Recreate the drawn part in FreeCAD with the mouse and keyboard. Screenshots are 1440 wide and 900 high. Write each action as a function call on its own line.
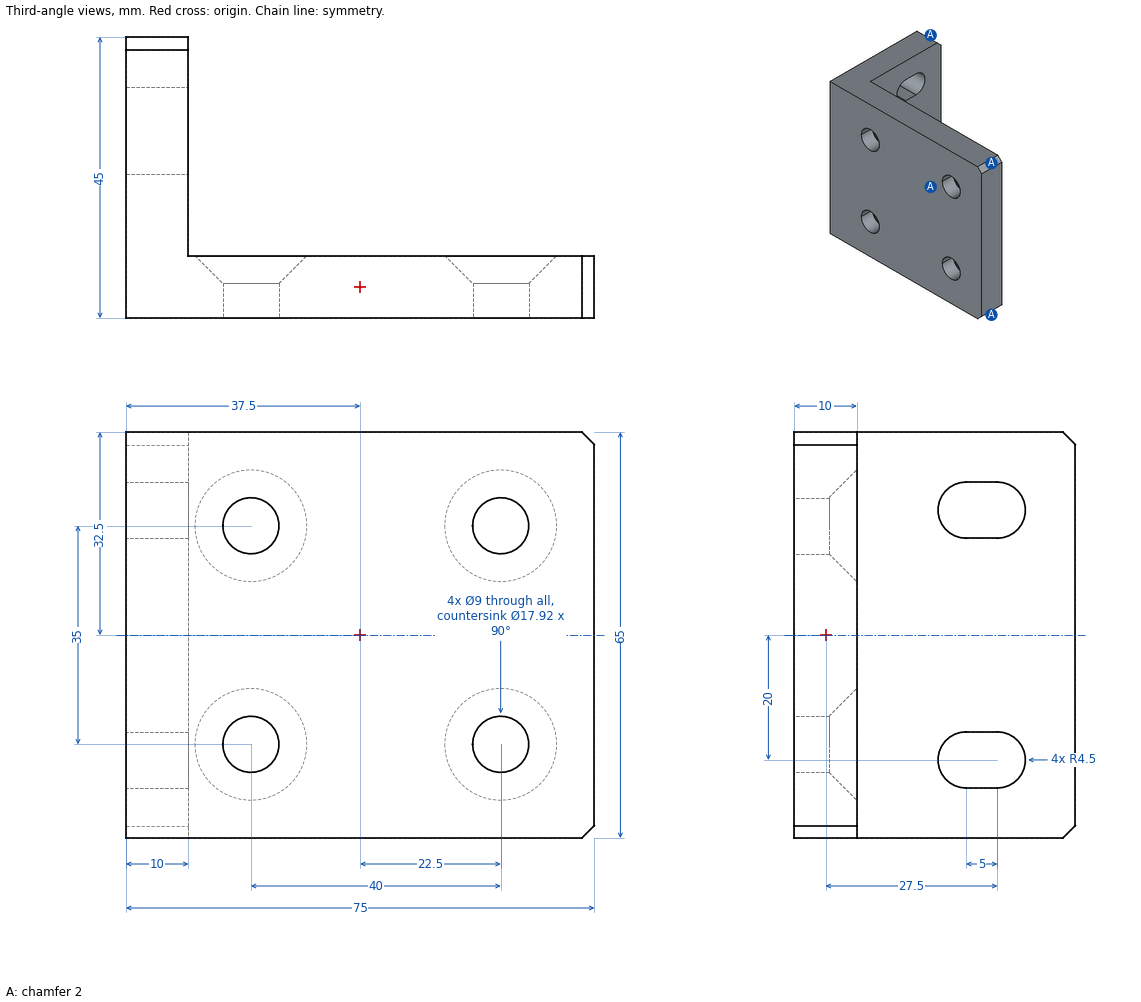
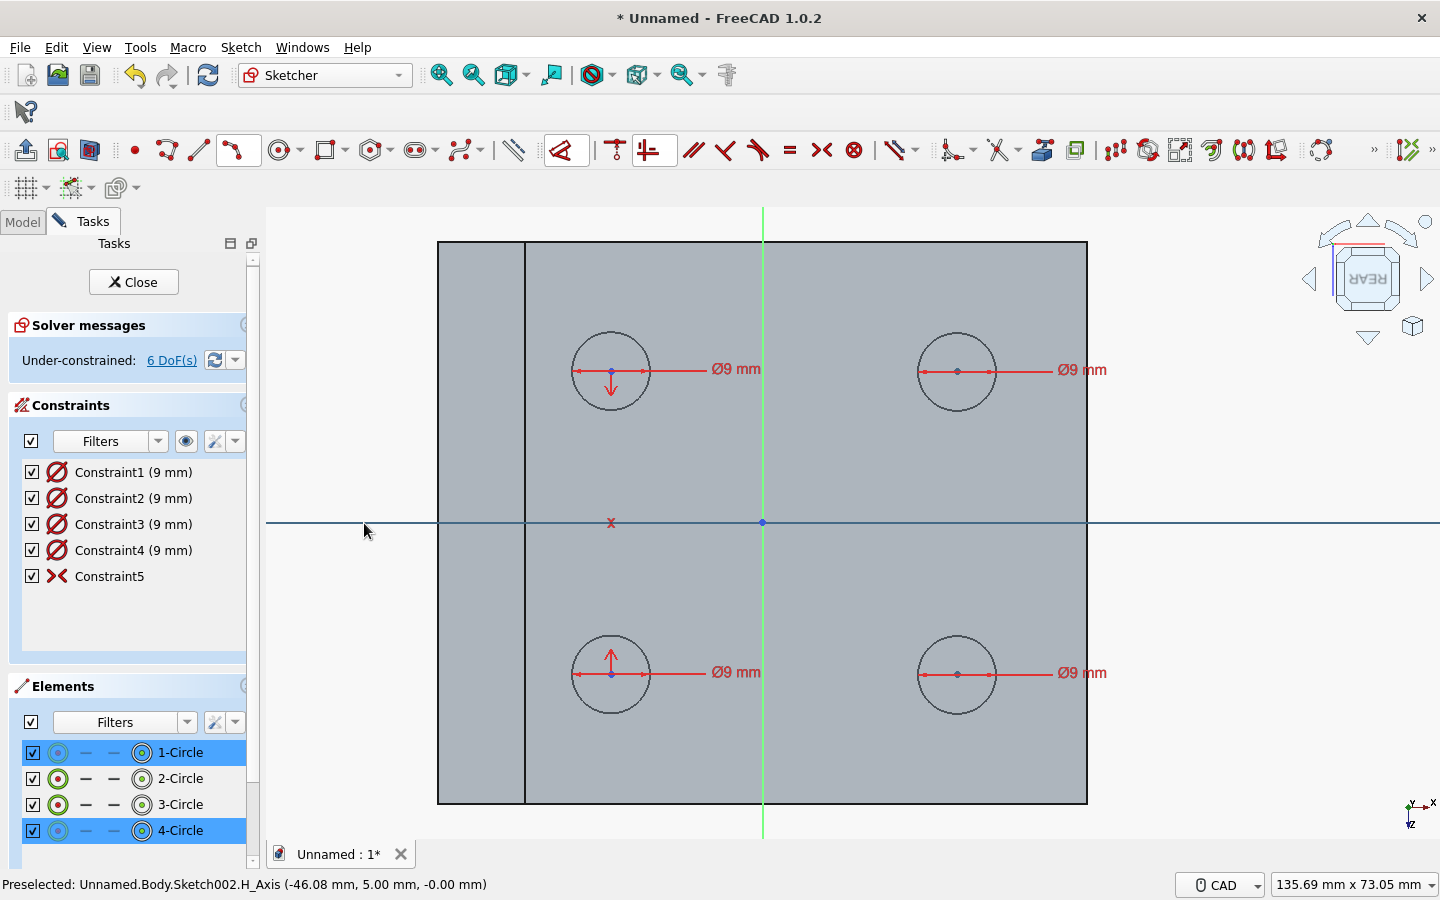
key(s)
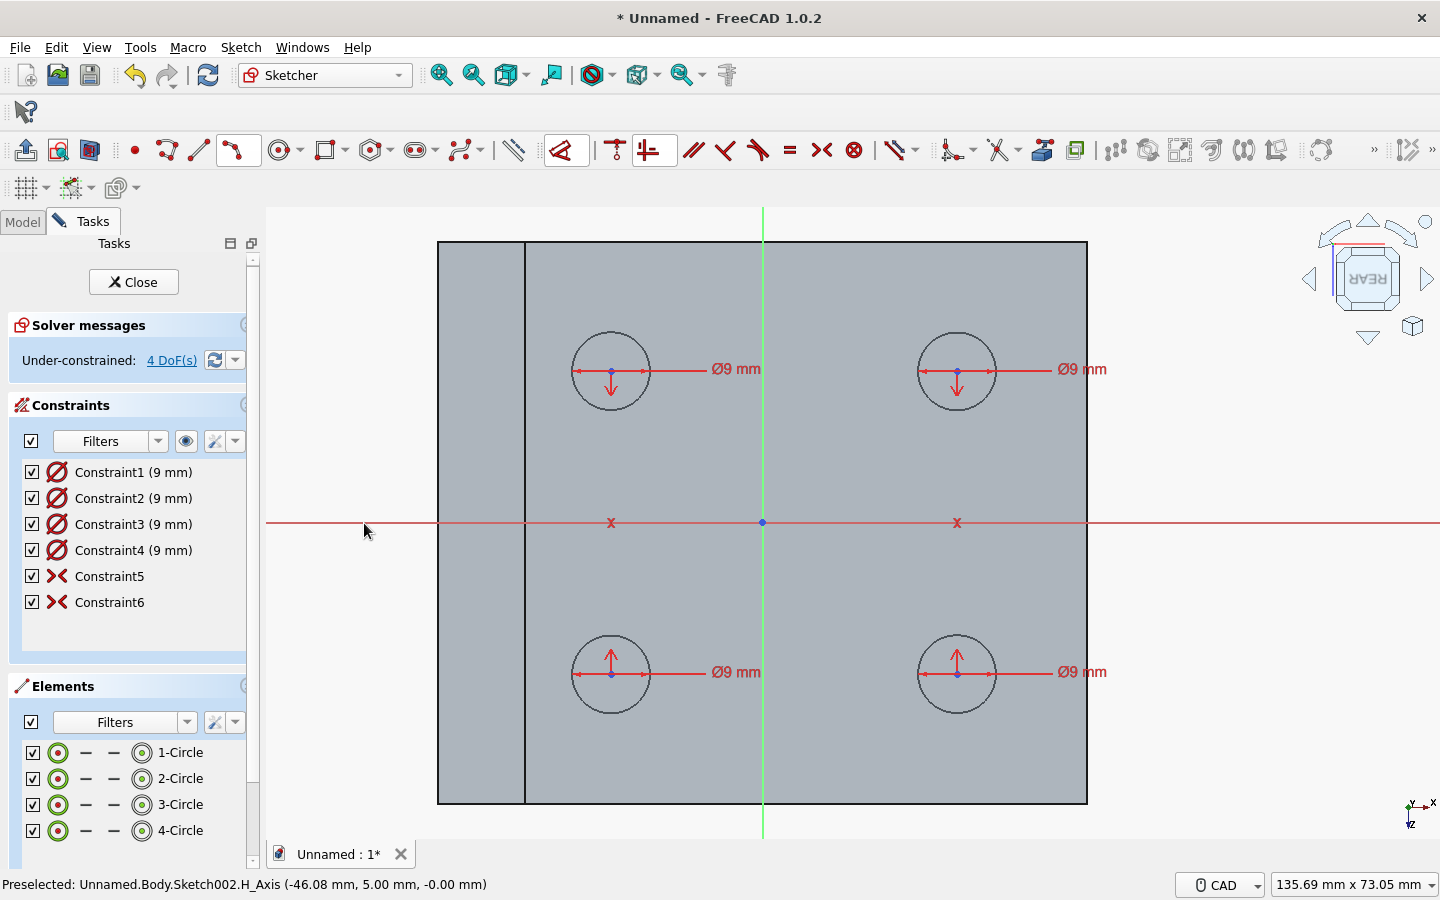
key(d)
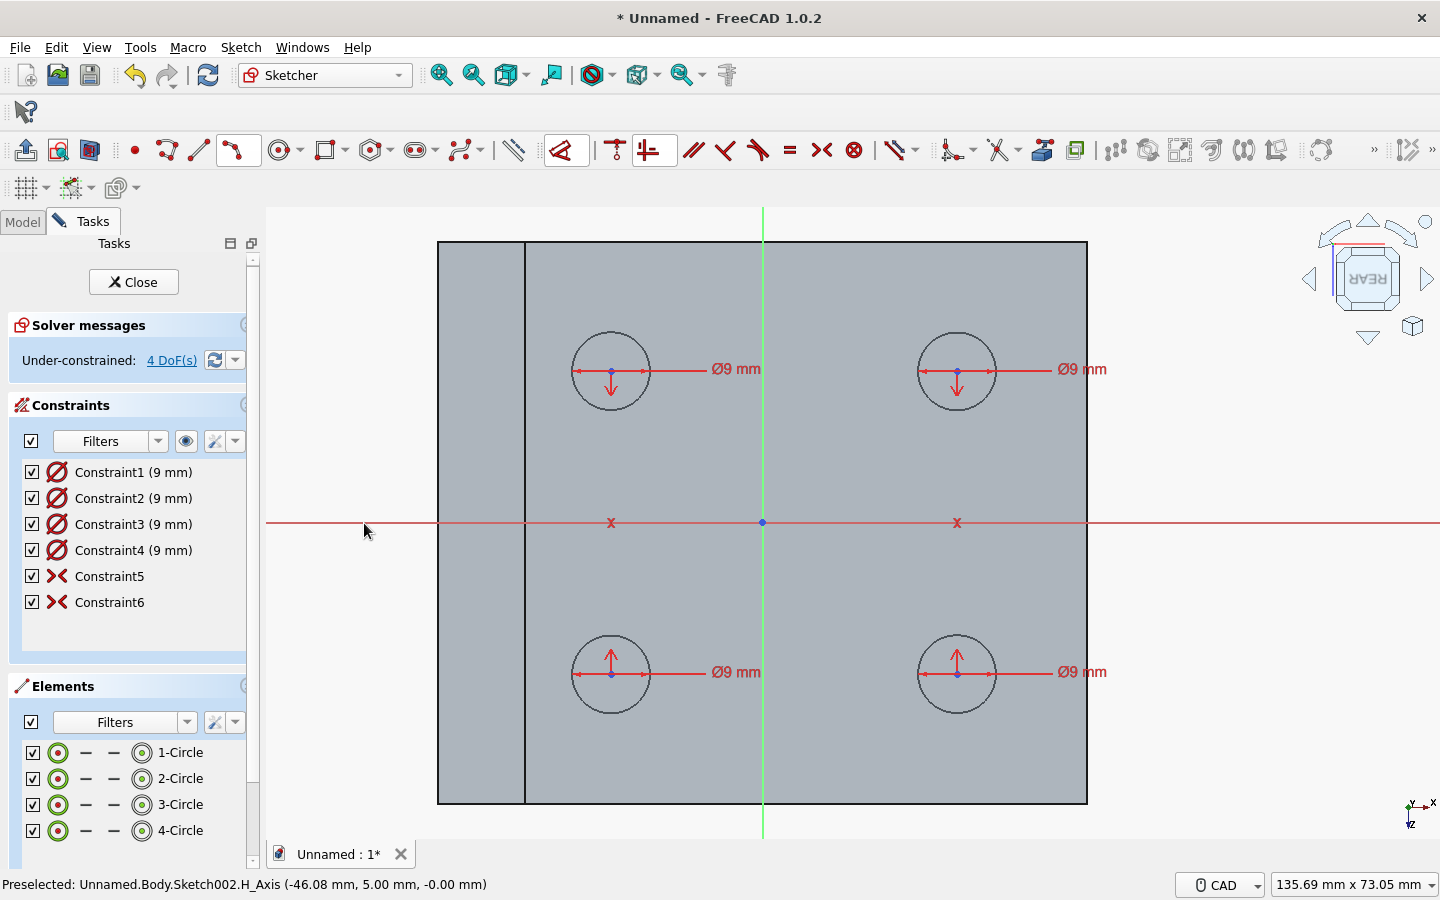
click(957, 371)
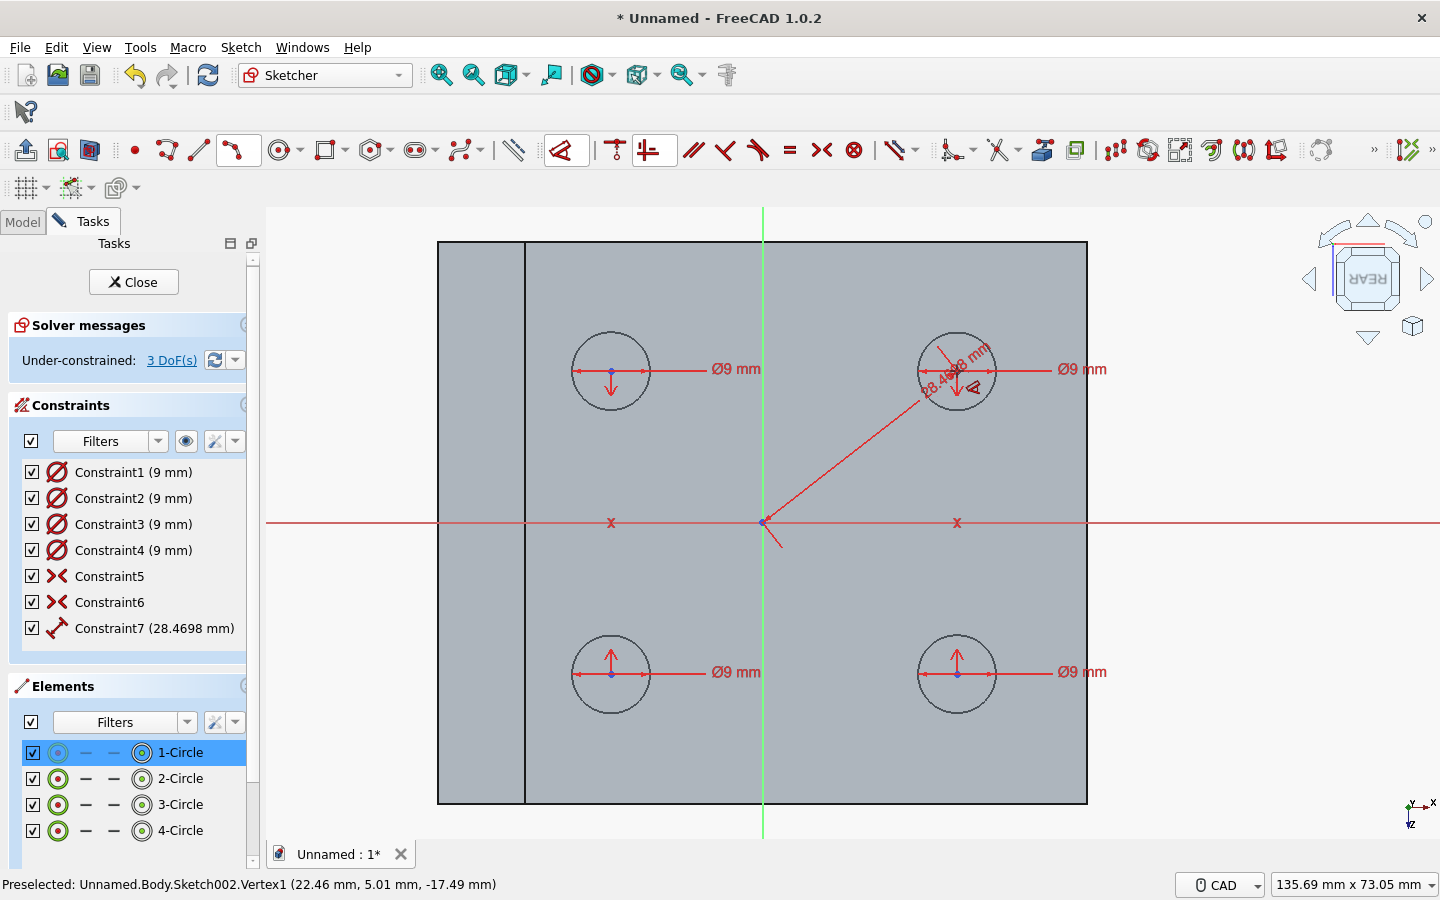
click(611, 371)
click(784, 337)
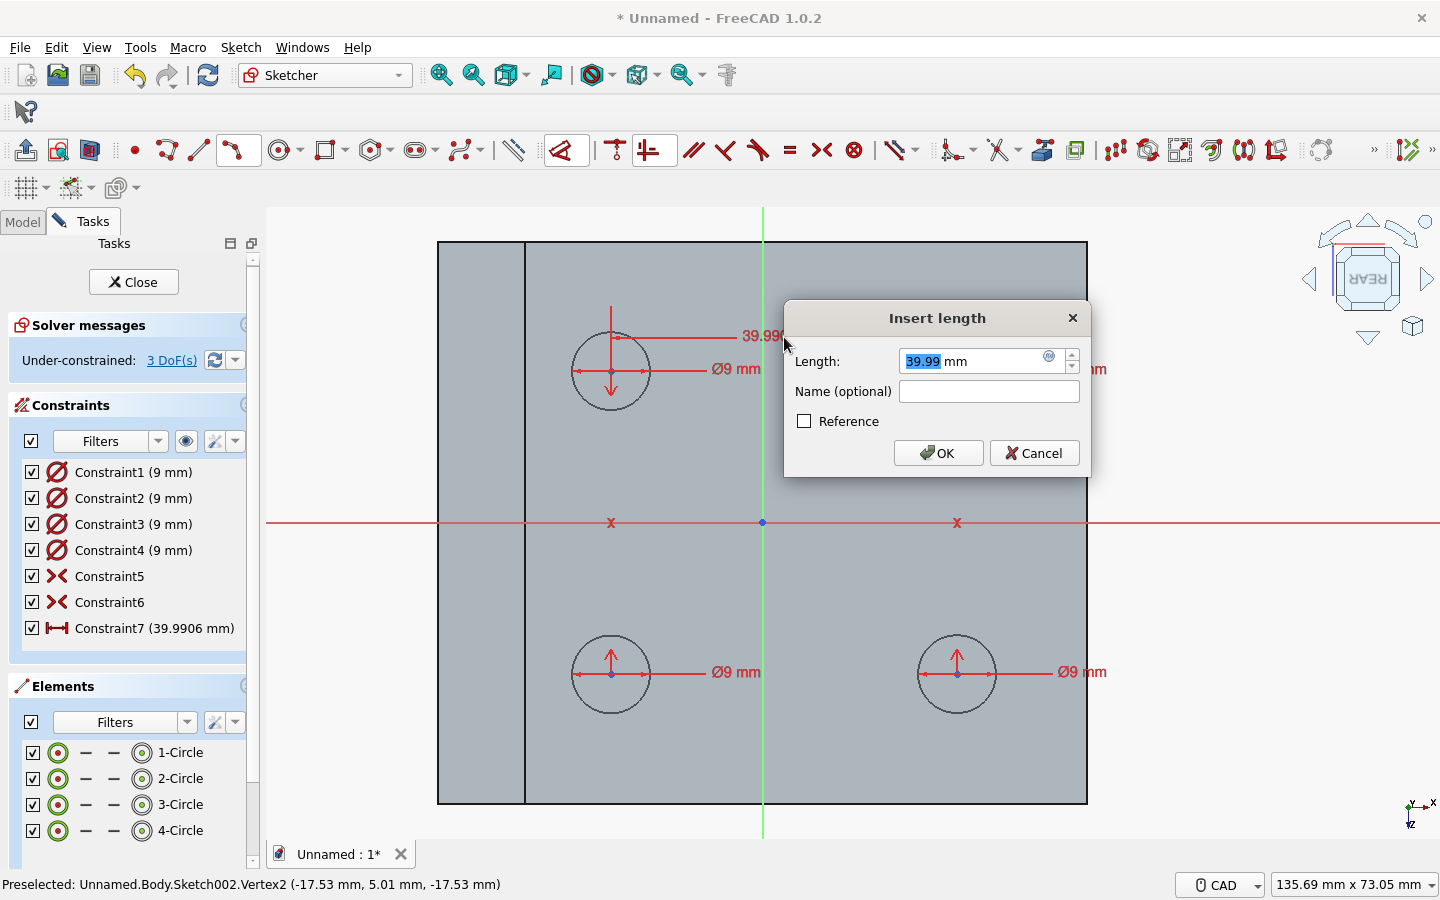
text(40)
key(Return)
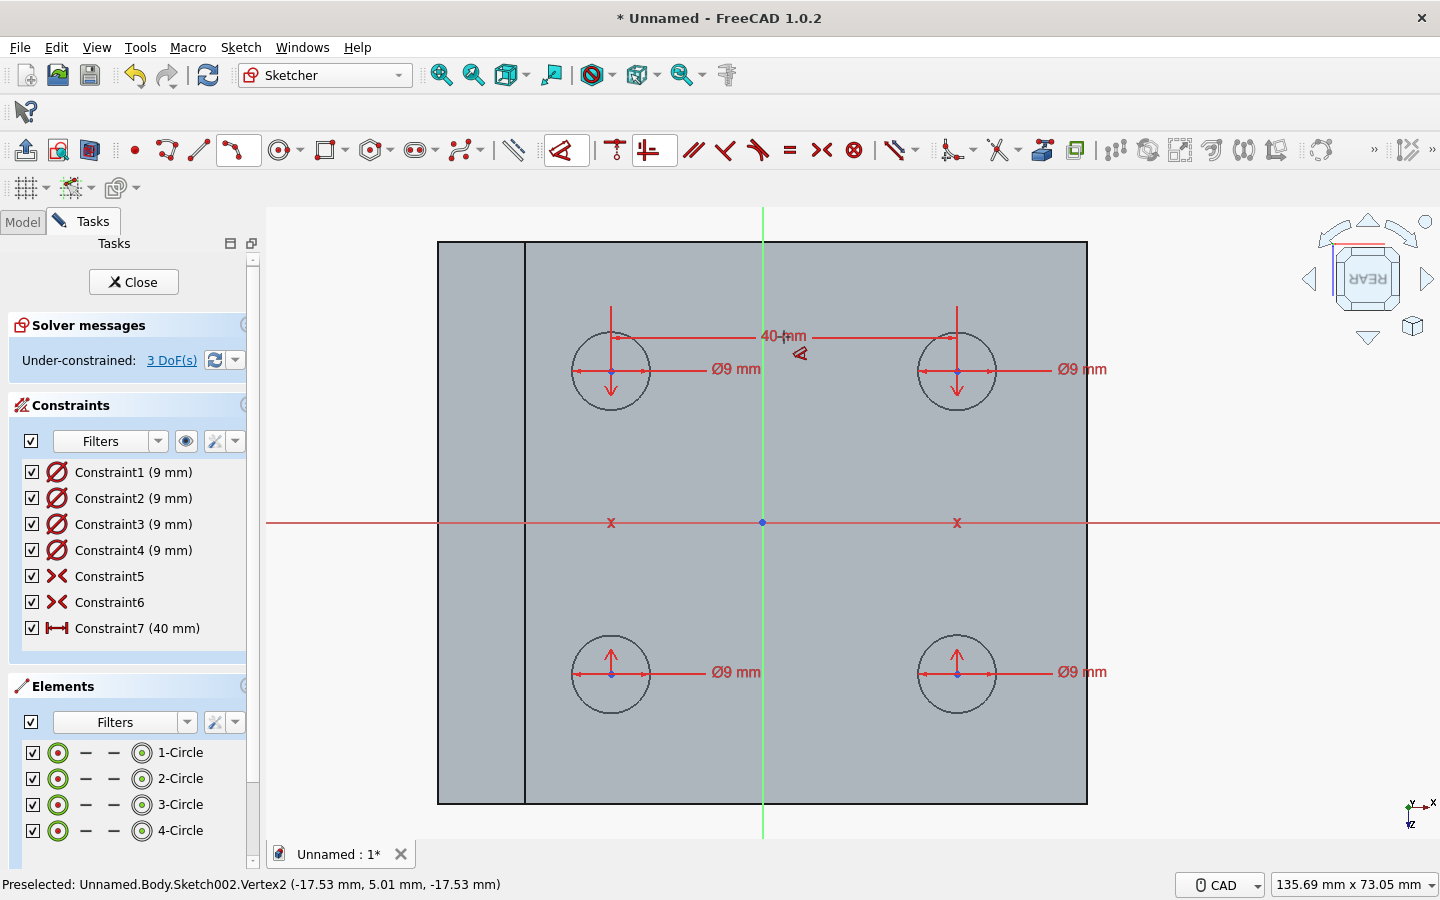
click(611, 371)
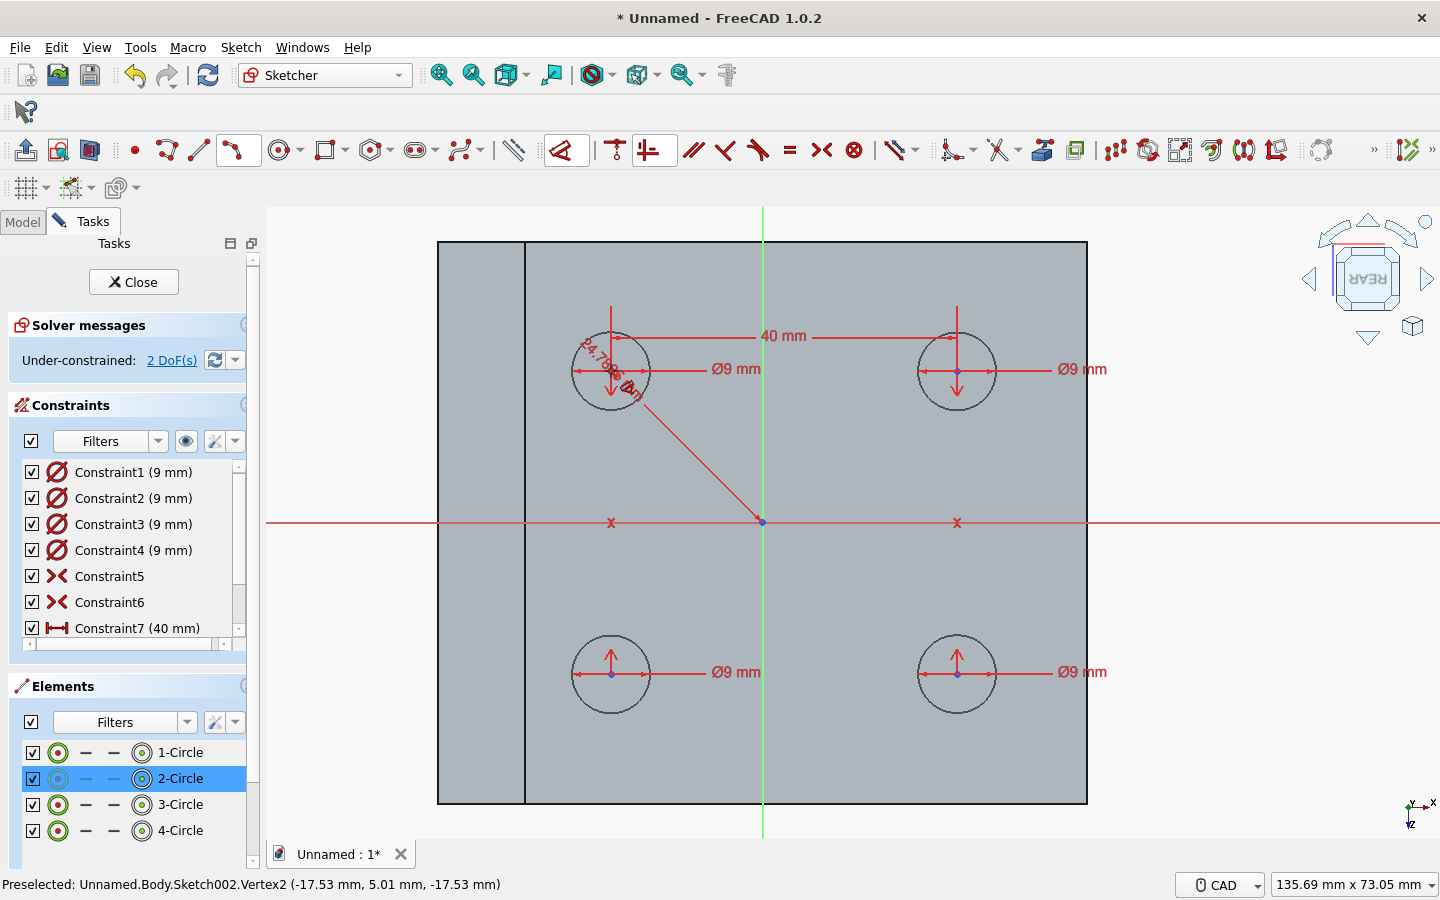
click(611, 674)
click(577, 453)